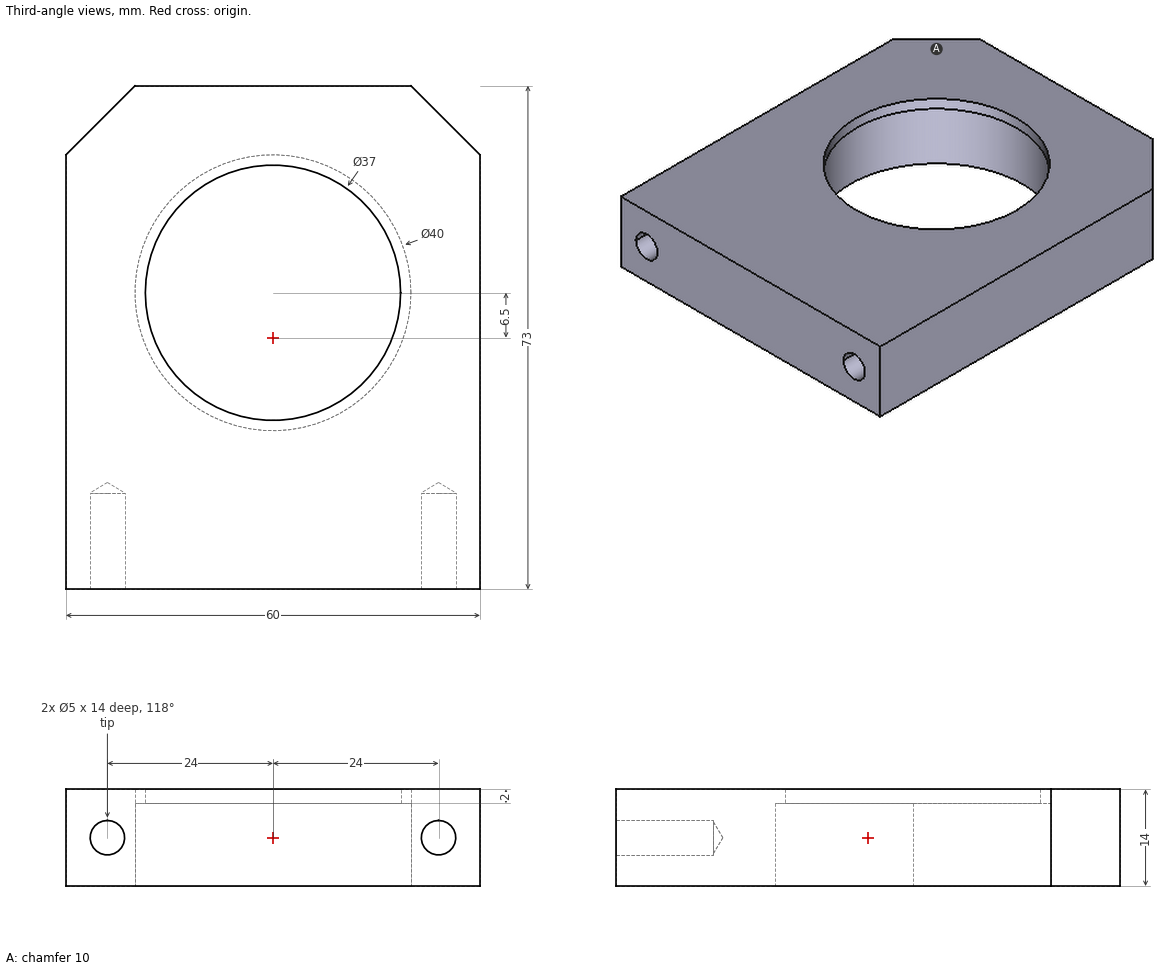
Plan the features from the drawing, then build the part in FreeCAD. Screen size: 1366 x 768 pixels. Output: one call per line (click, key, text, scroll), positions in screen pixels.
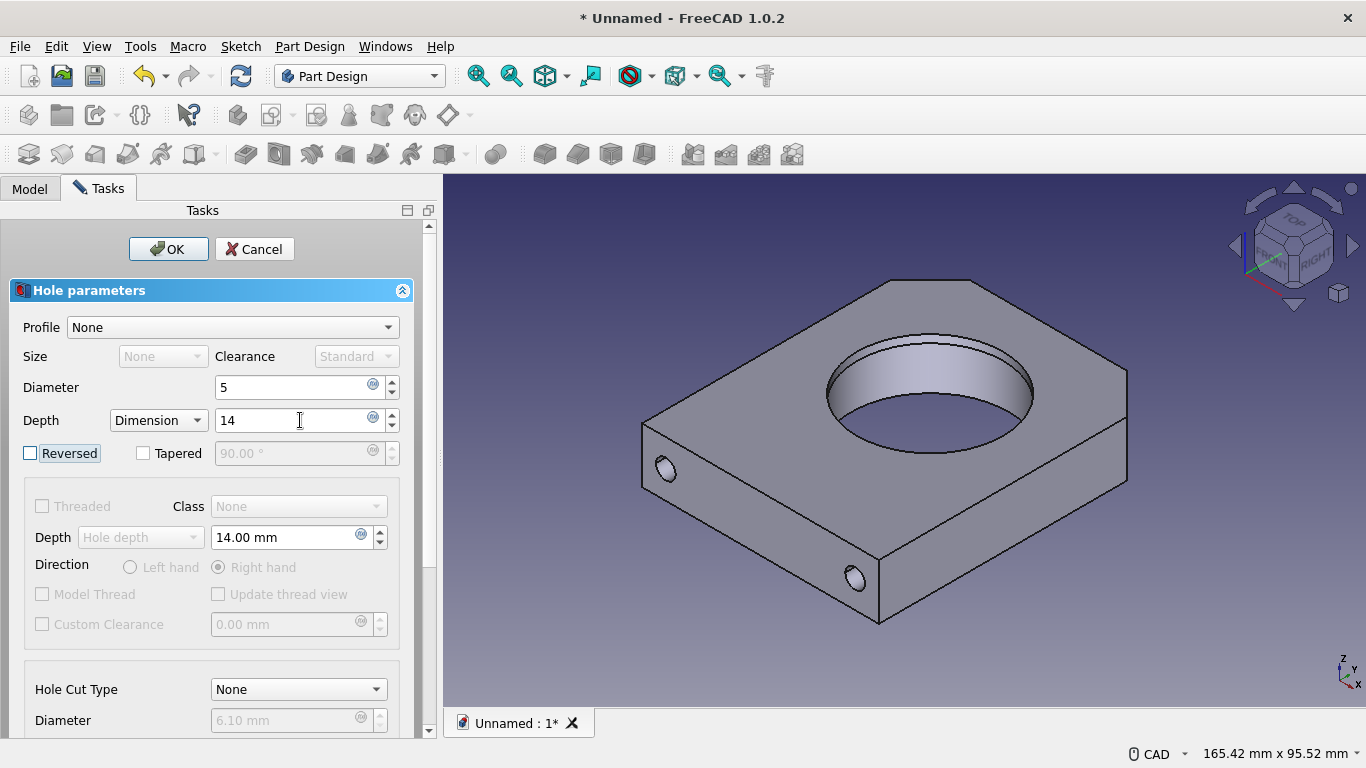
click(169, 249)